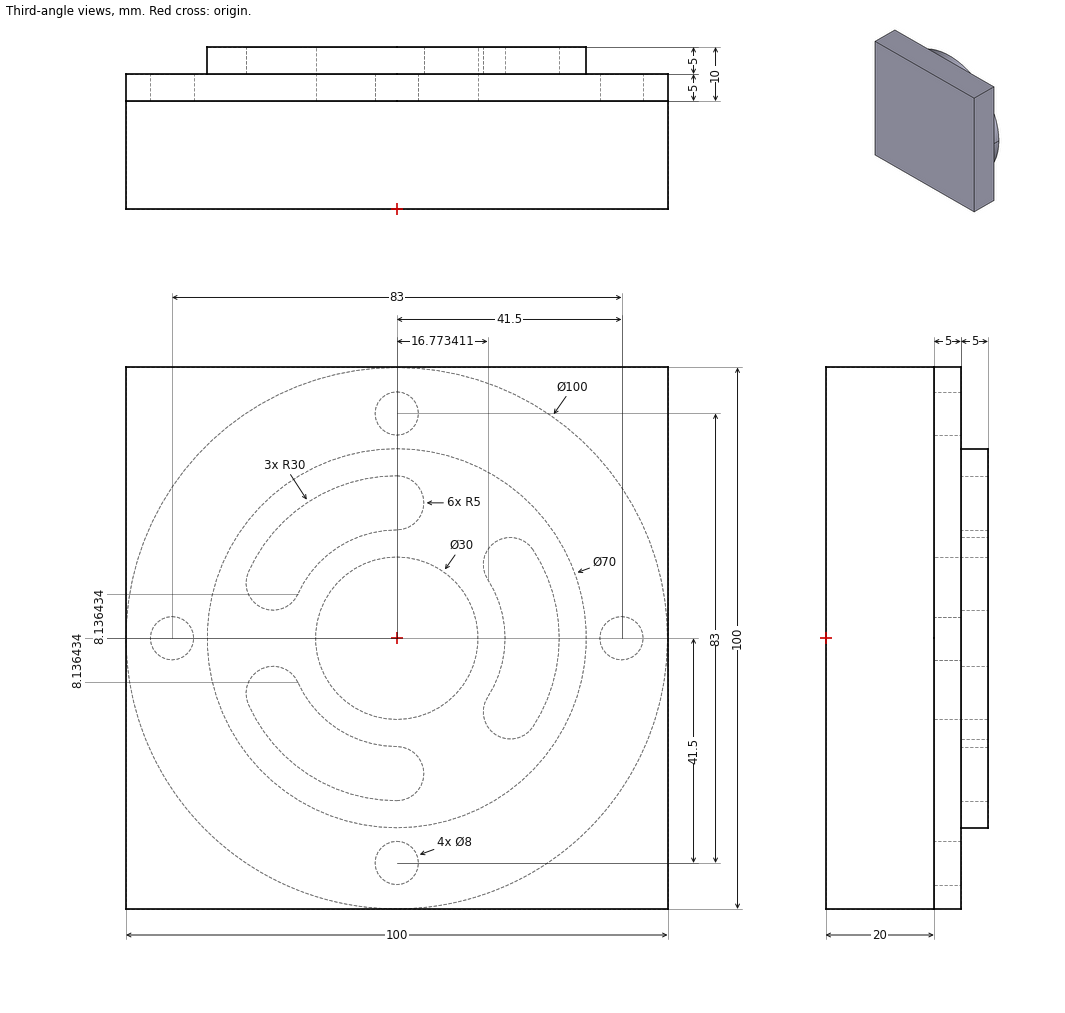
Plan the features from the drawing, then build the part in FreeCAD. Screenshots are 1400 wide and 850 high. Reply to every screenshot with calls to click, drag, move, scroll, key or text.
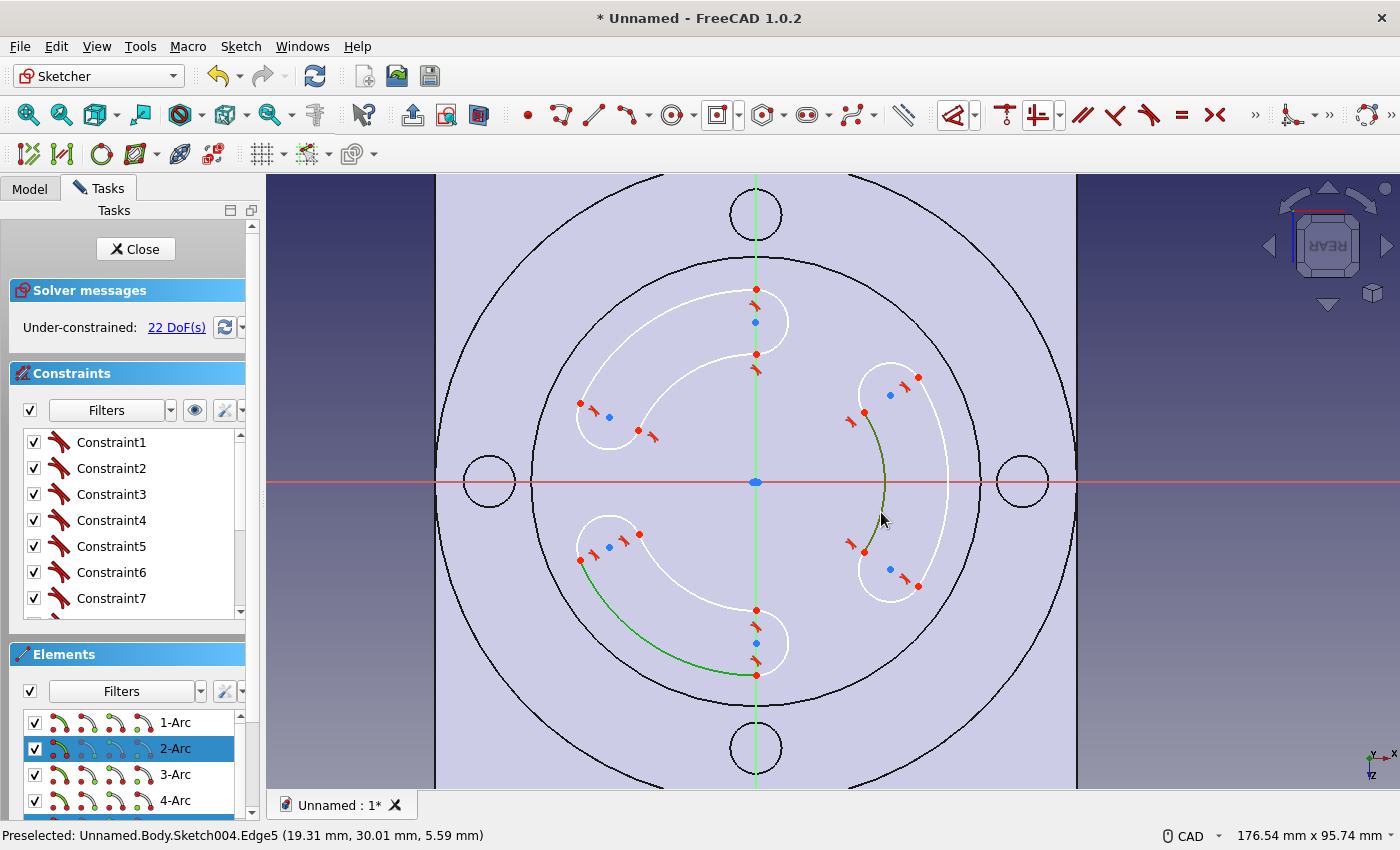
click(1005, 116)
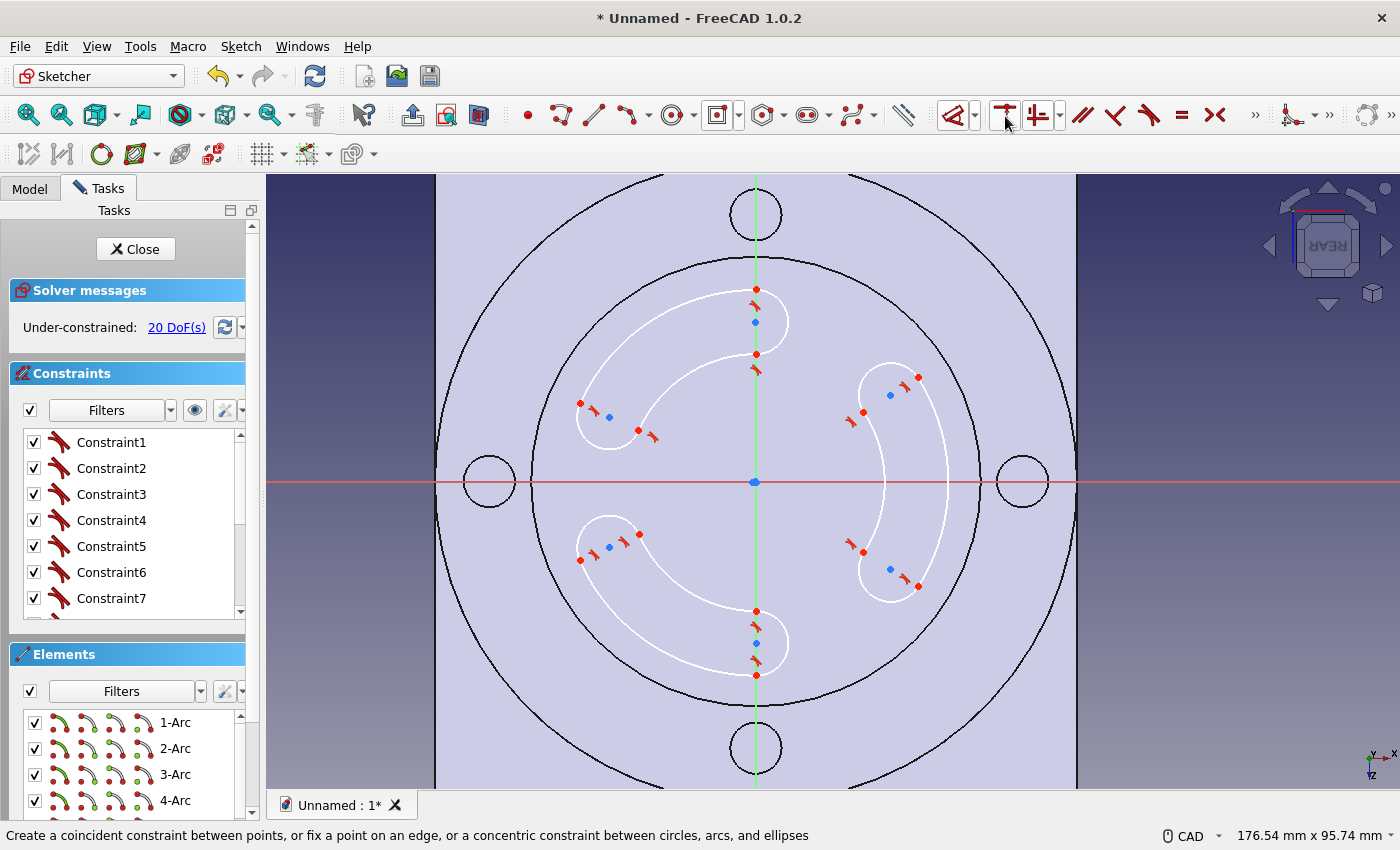
click(617, 616)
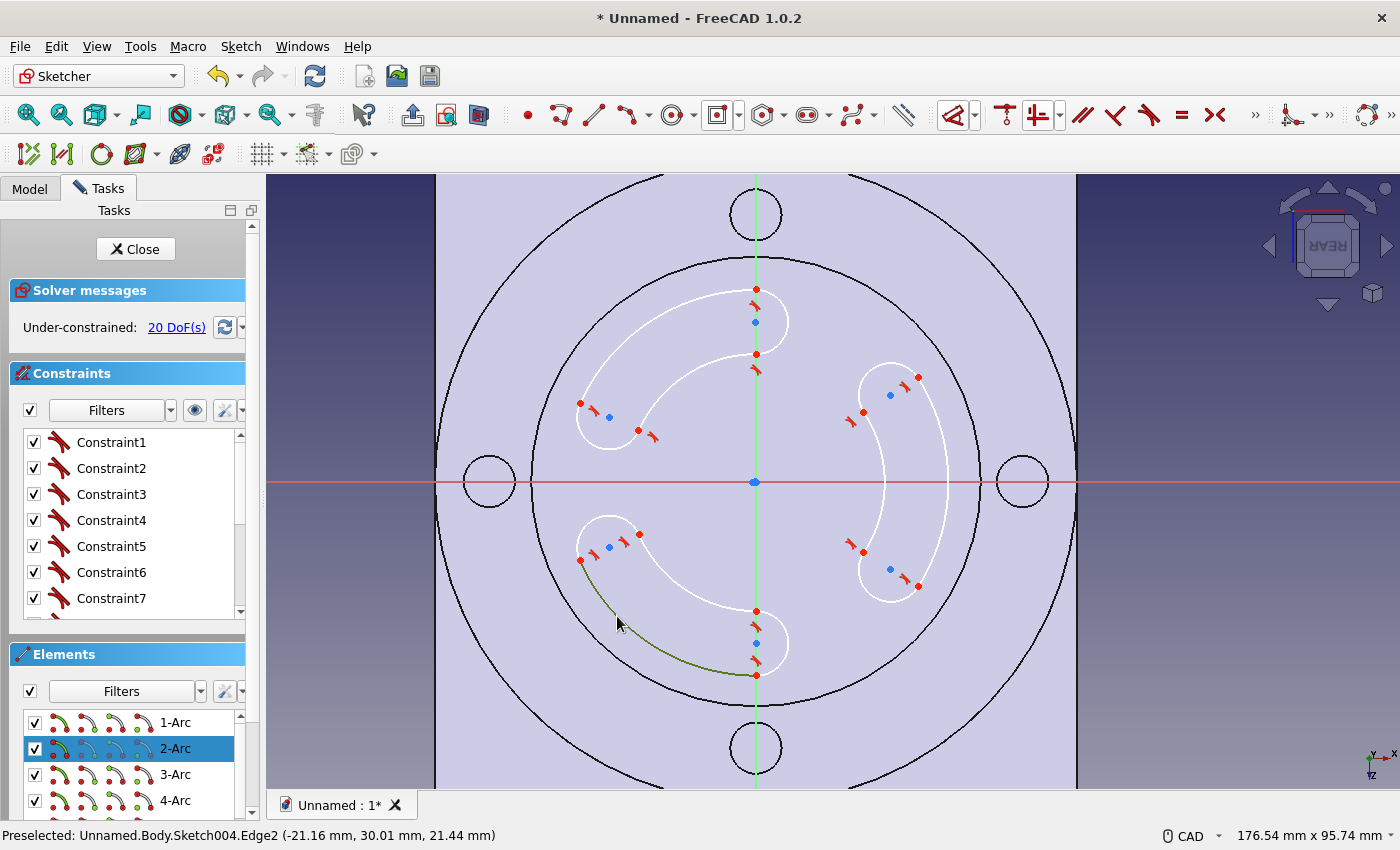
click(943, 526)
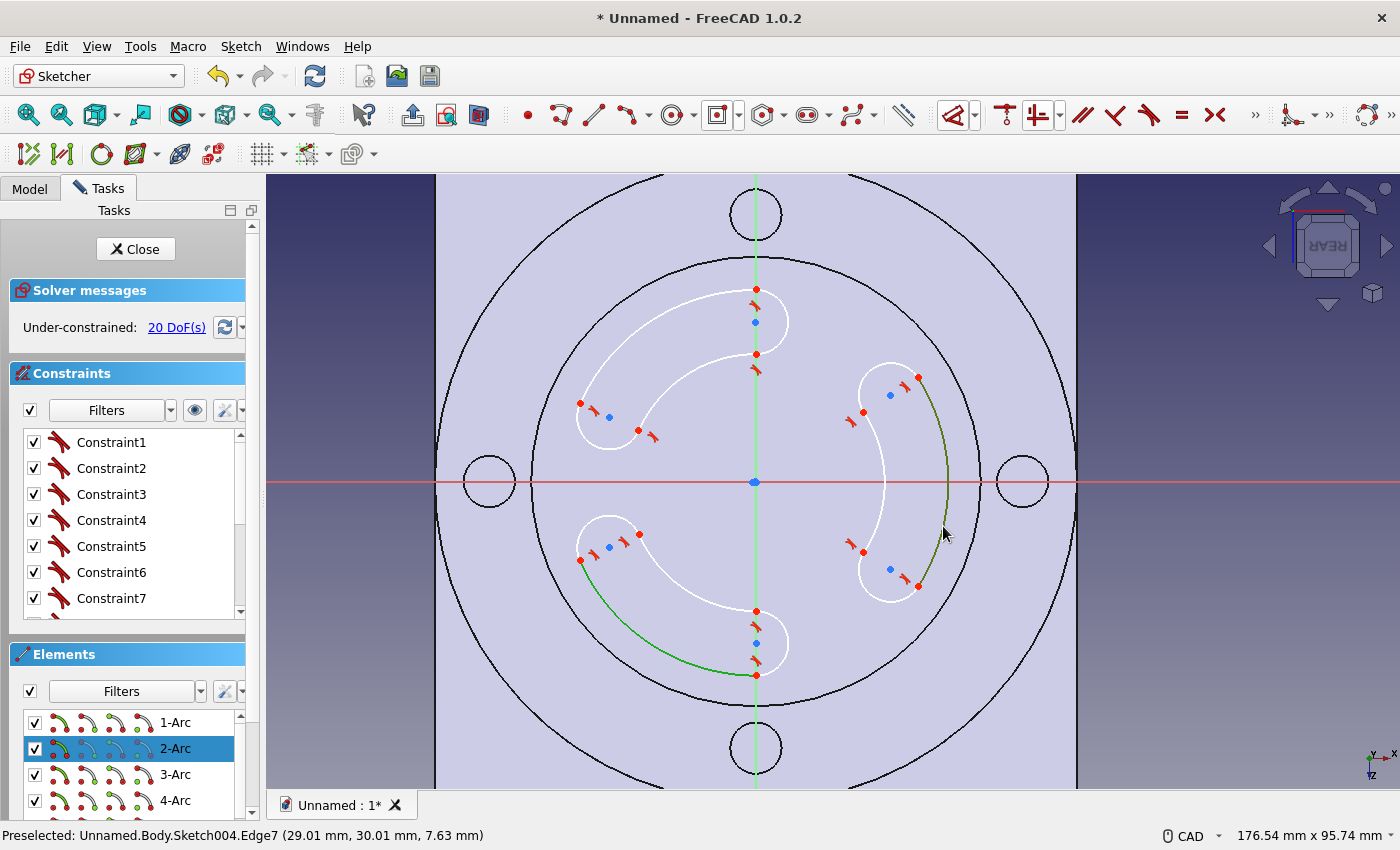
click(1005, 116)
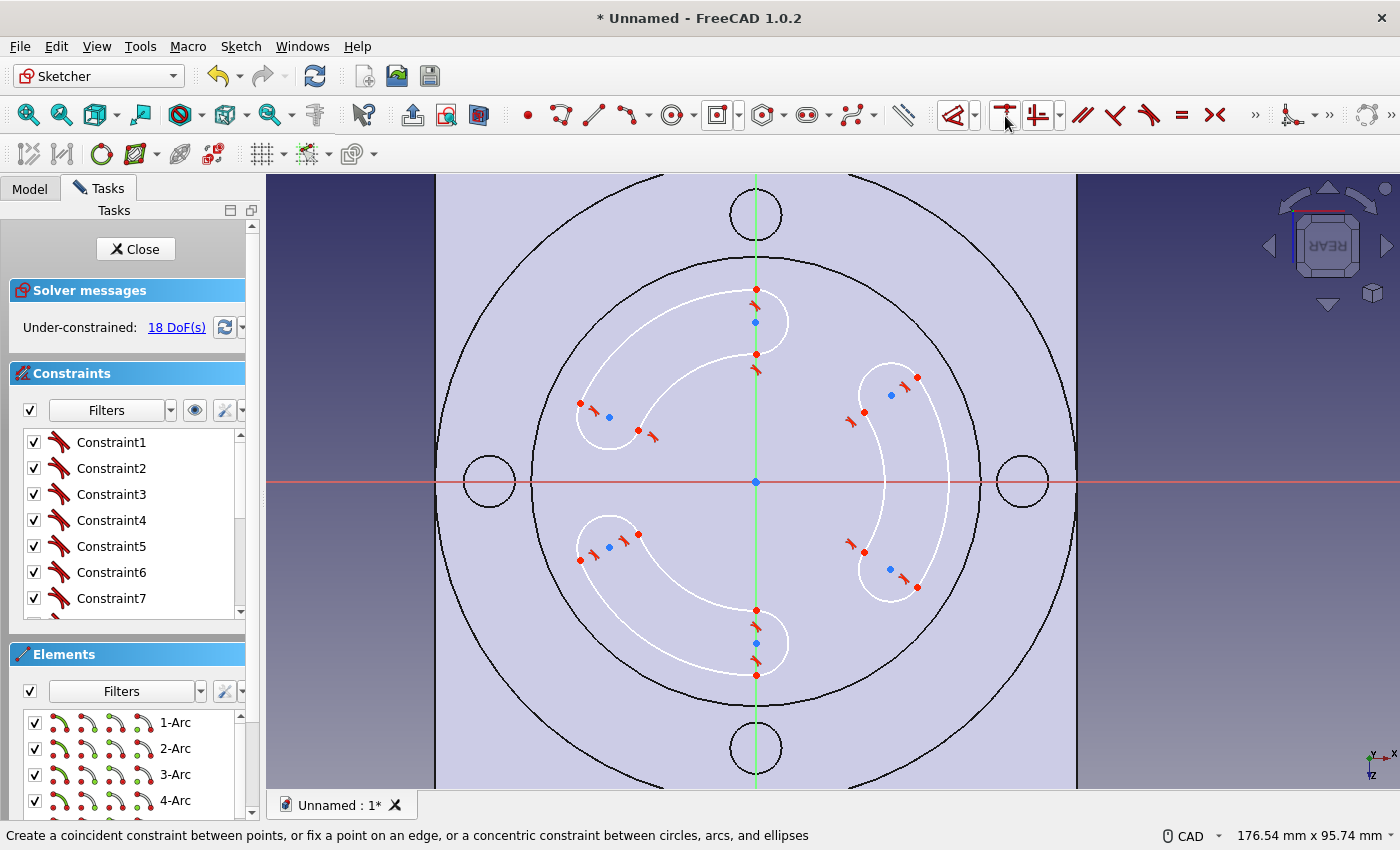
click(617, 616)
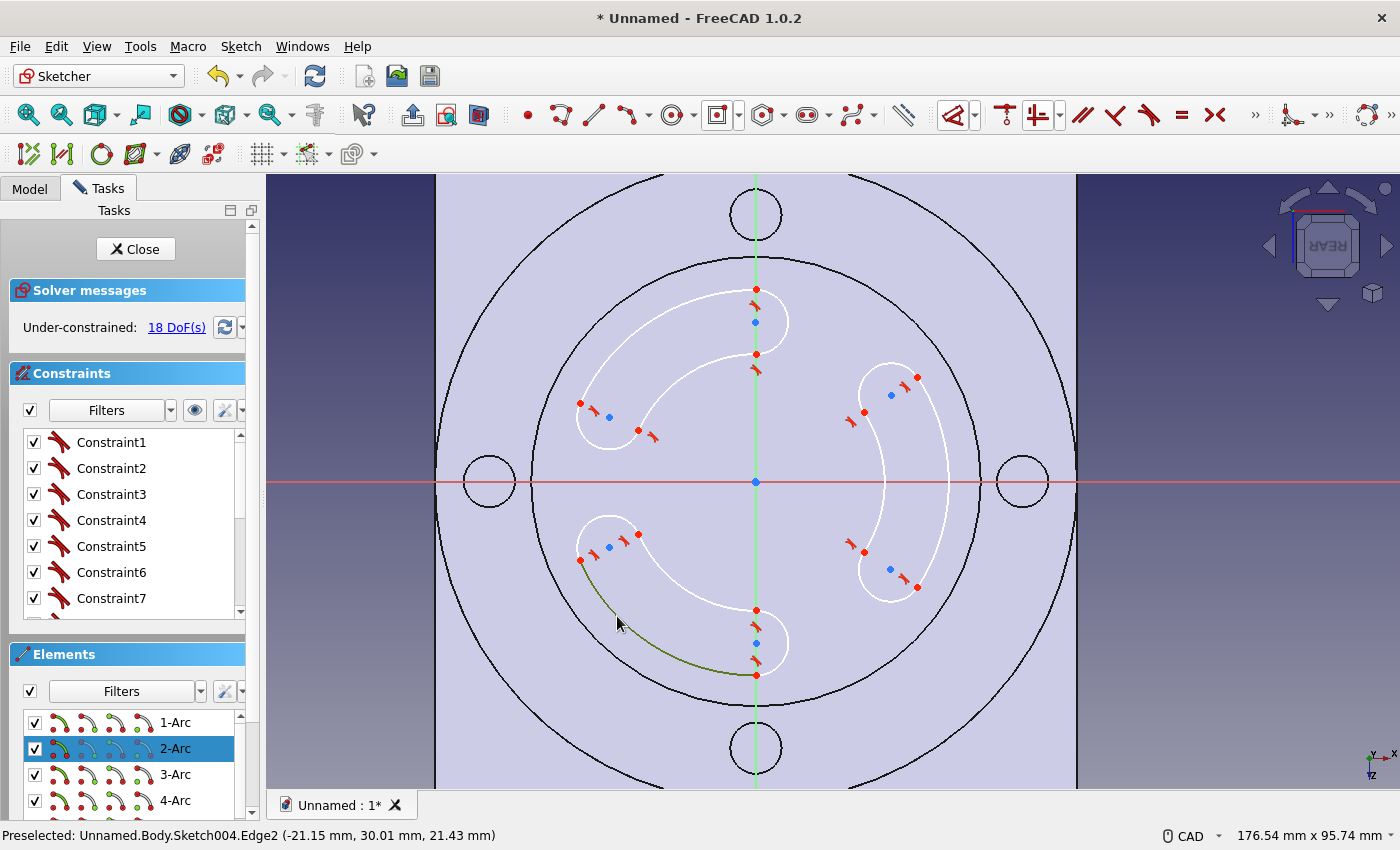
click(713, 362)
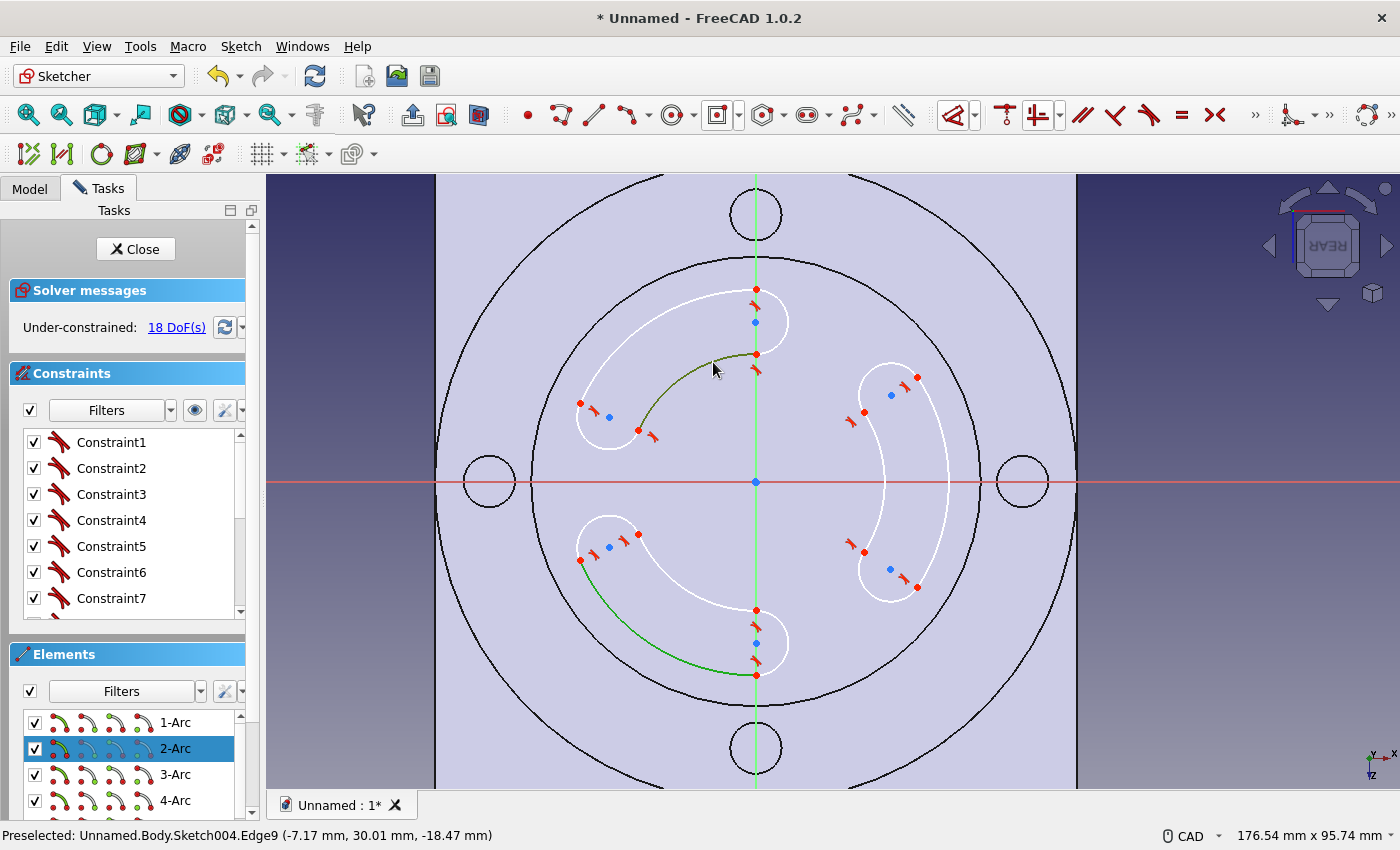
click(1005, 116)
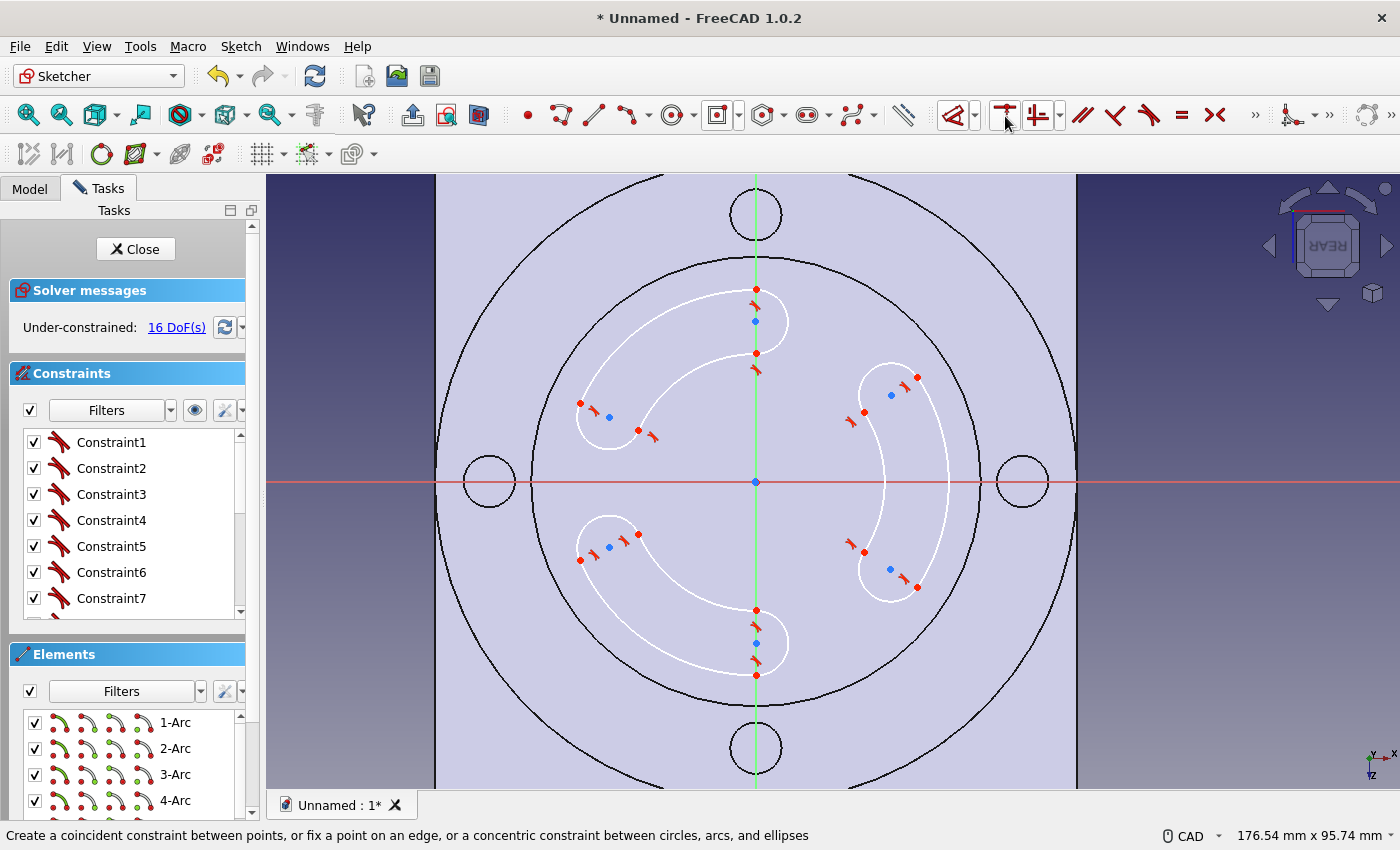
click(617, 616)